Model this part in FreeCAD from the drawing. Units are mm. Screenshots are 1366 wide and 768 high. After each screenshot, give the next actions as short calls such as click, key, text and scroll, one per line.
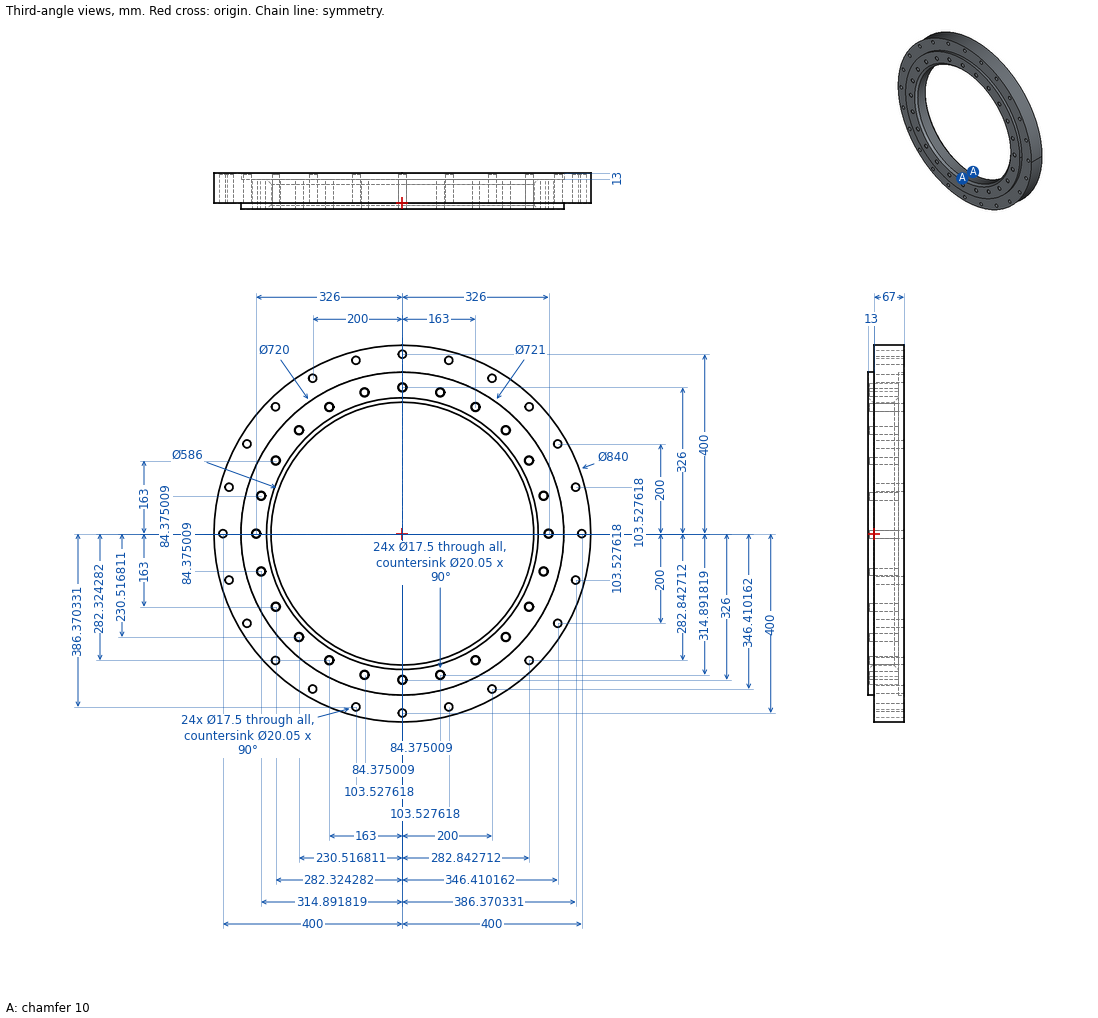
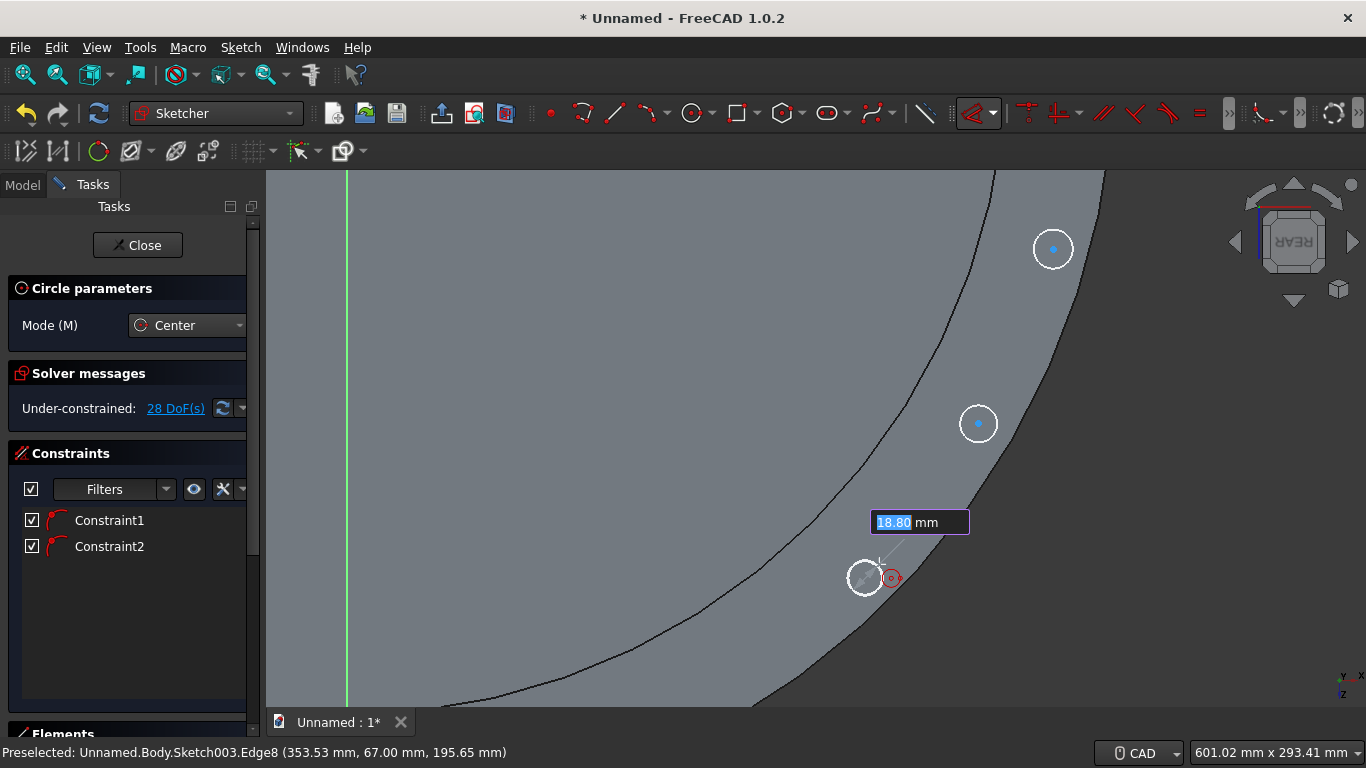
click(876, 561)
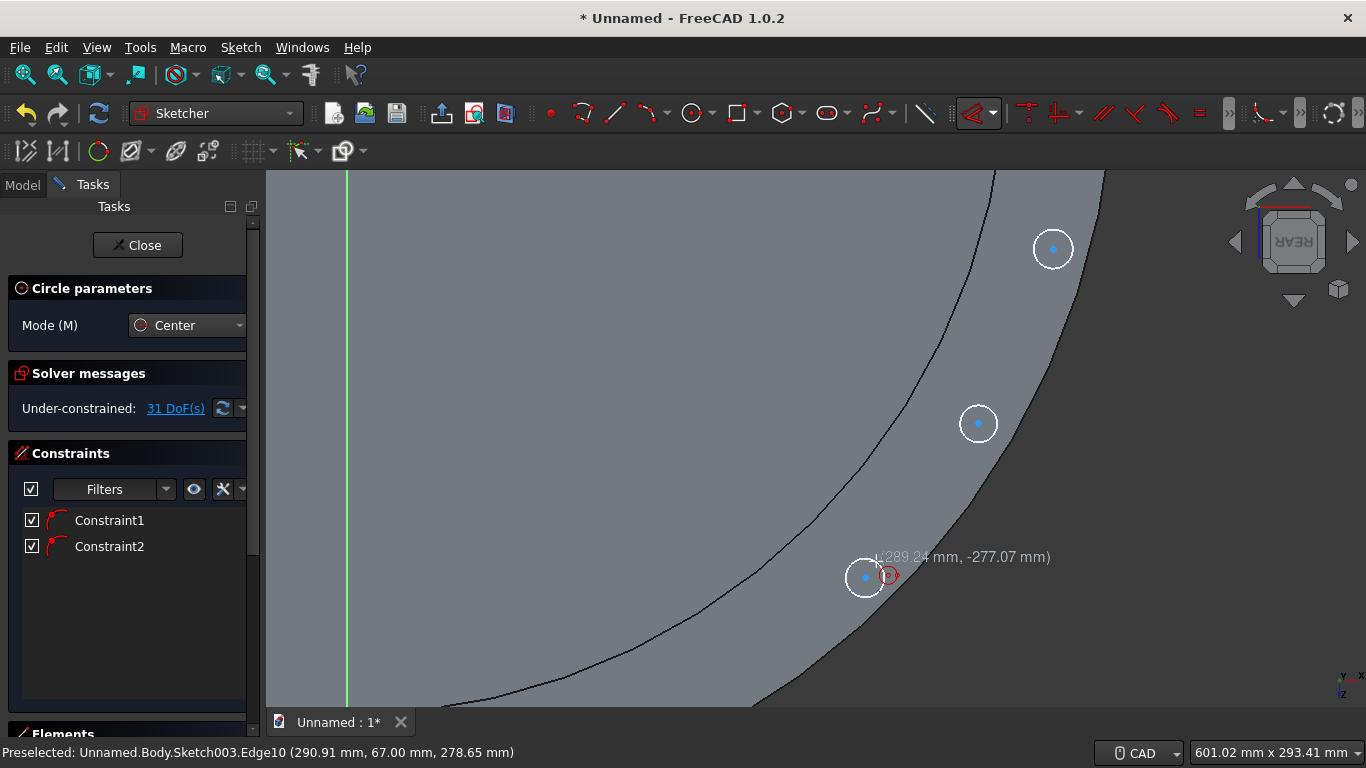
scroll(879, 564, down, 7)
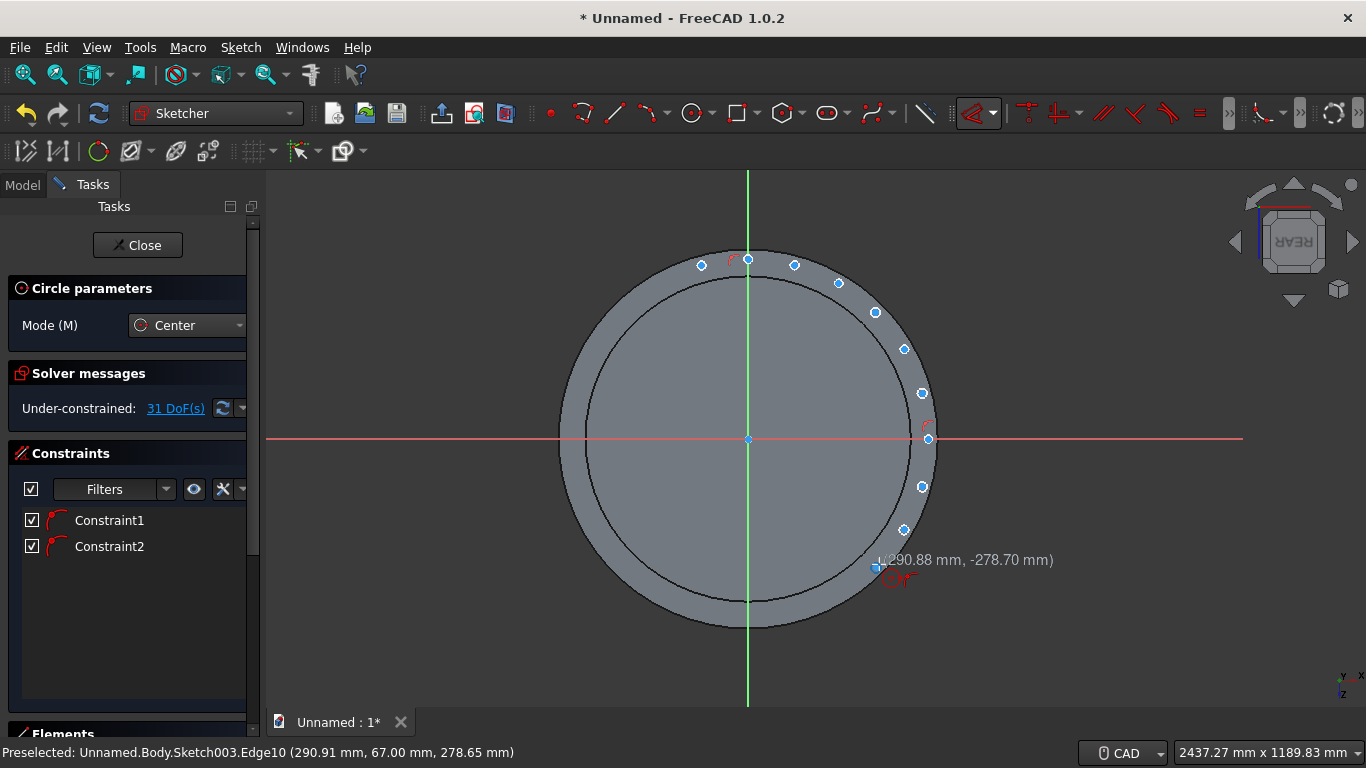
scroll(838, 595, up, 9)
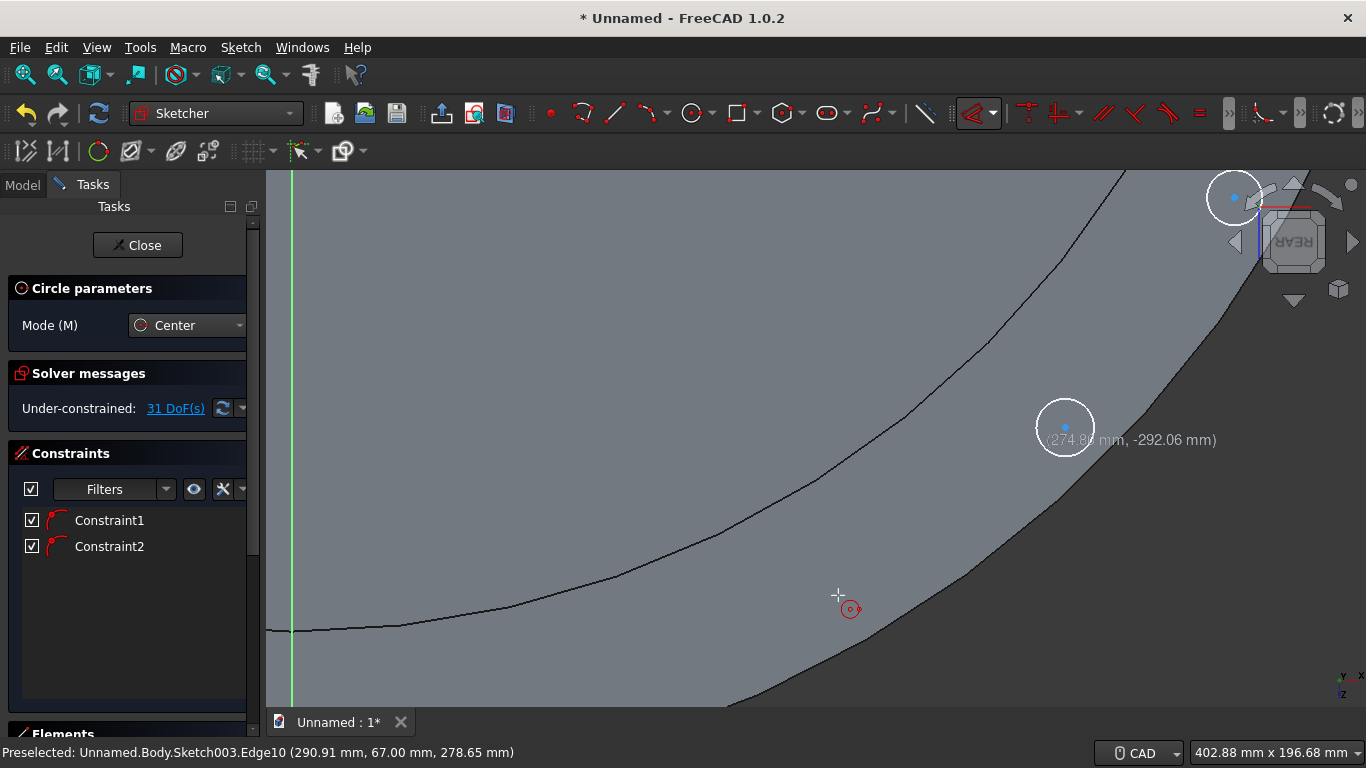
scroll(838, 595, down, 9)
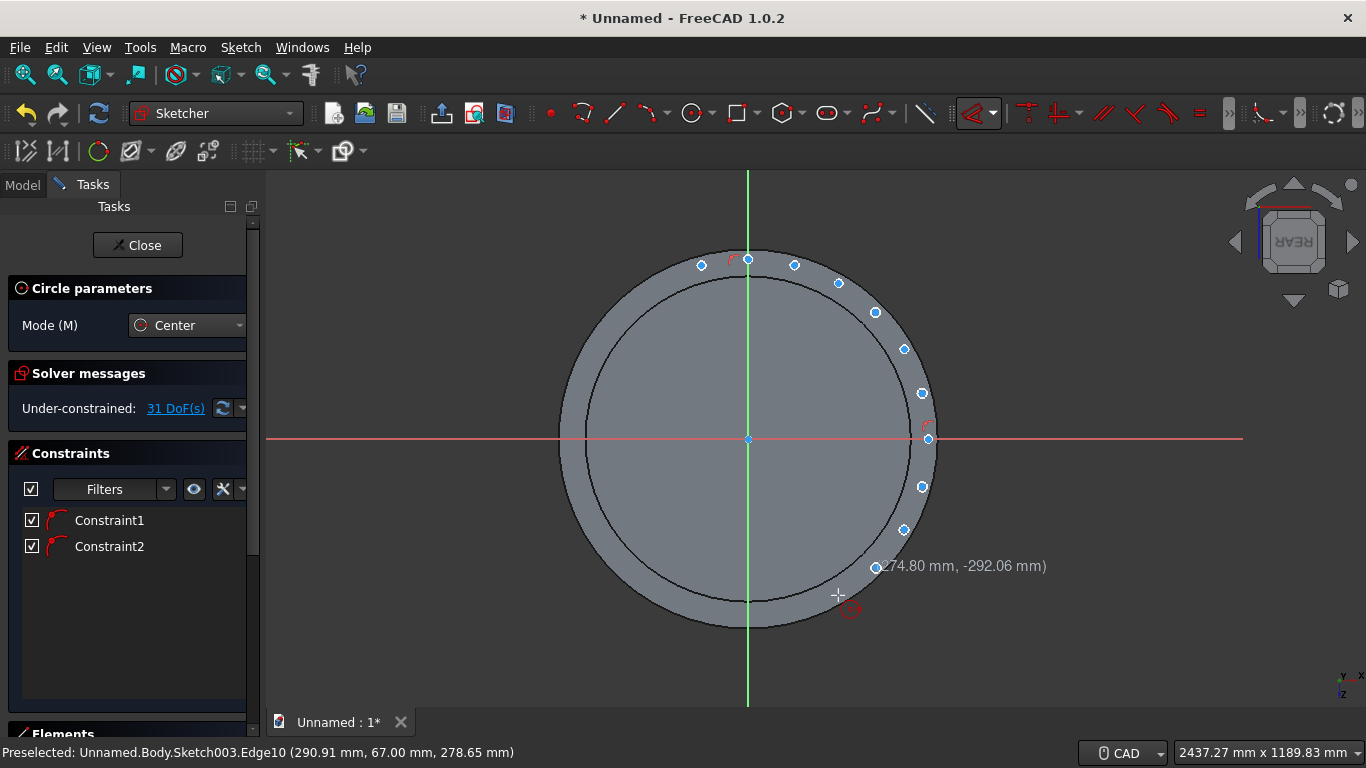
click(838, 595)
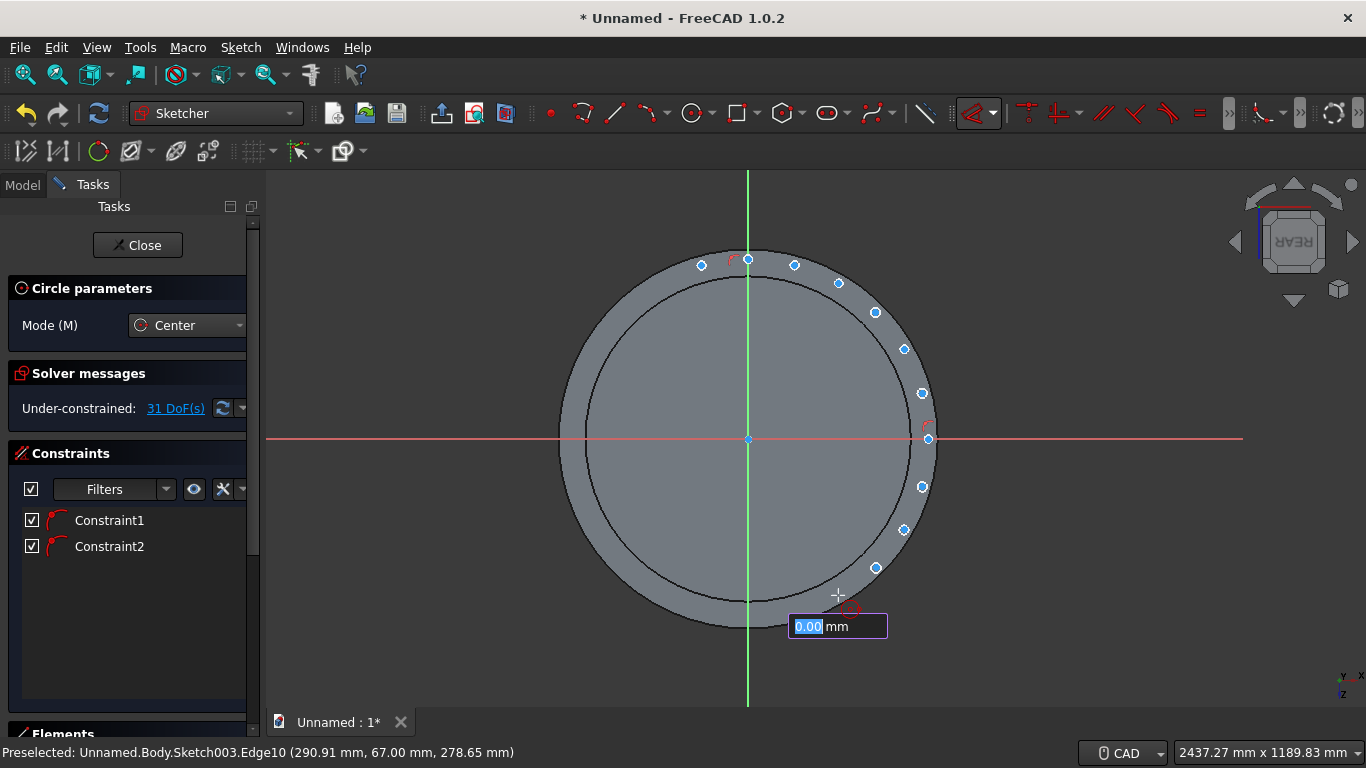
scroll(841, 593, up, 7)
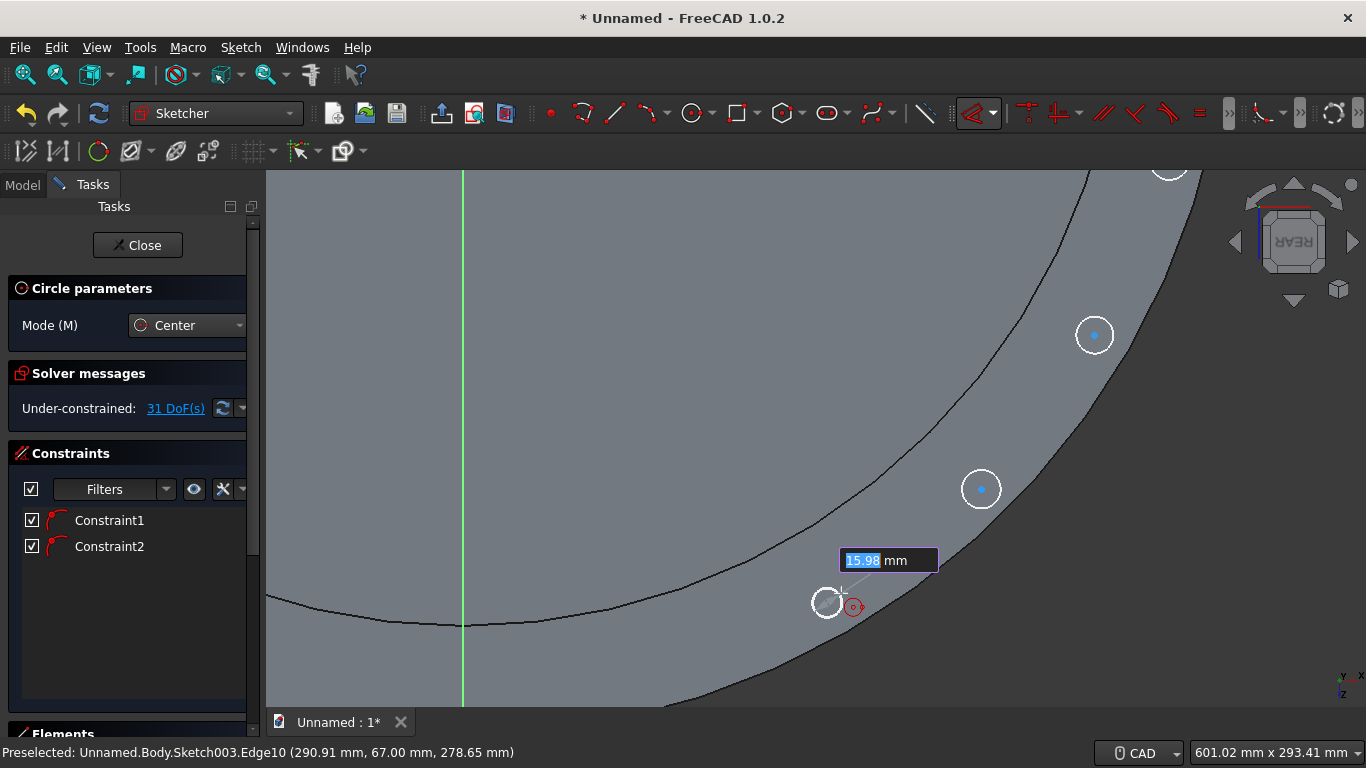
click(840, 589)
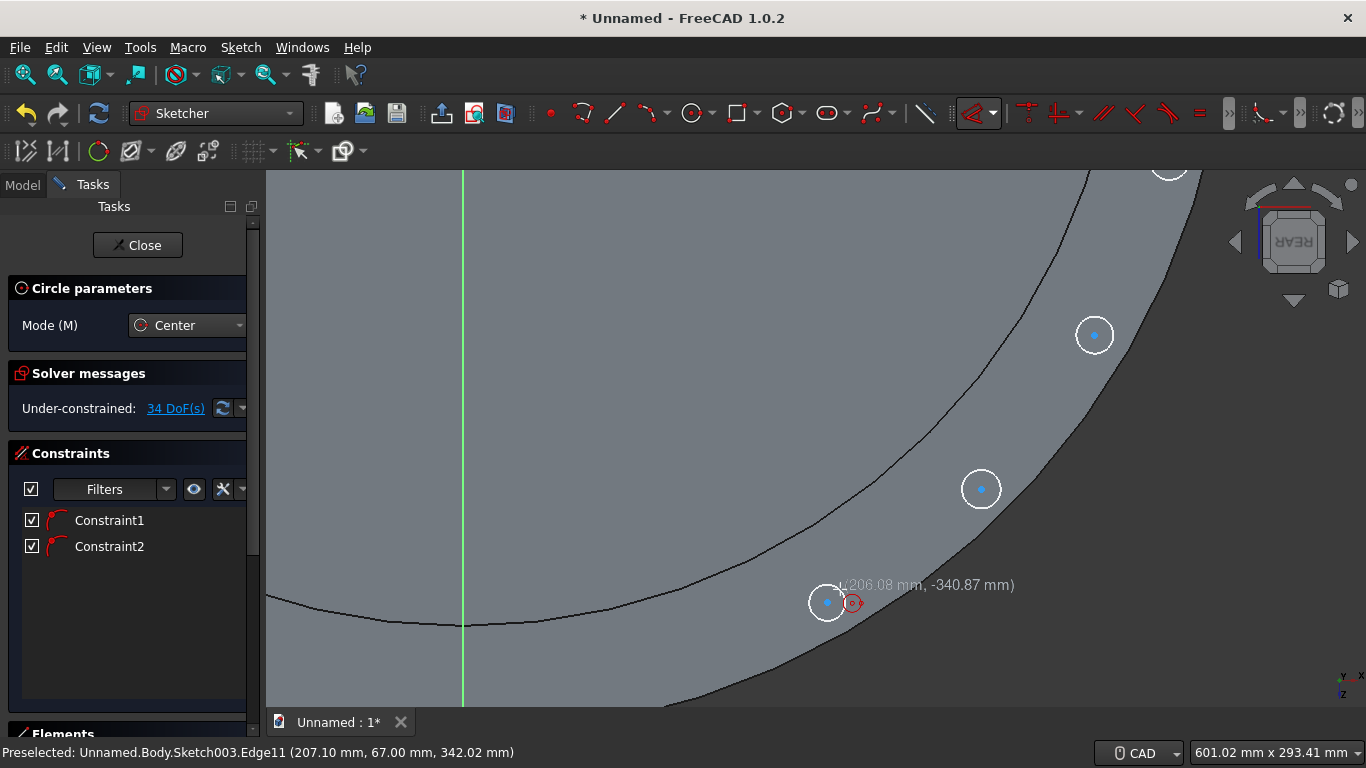
scroll(652, 673, up, 2)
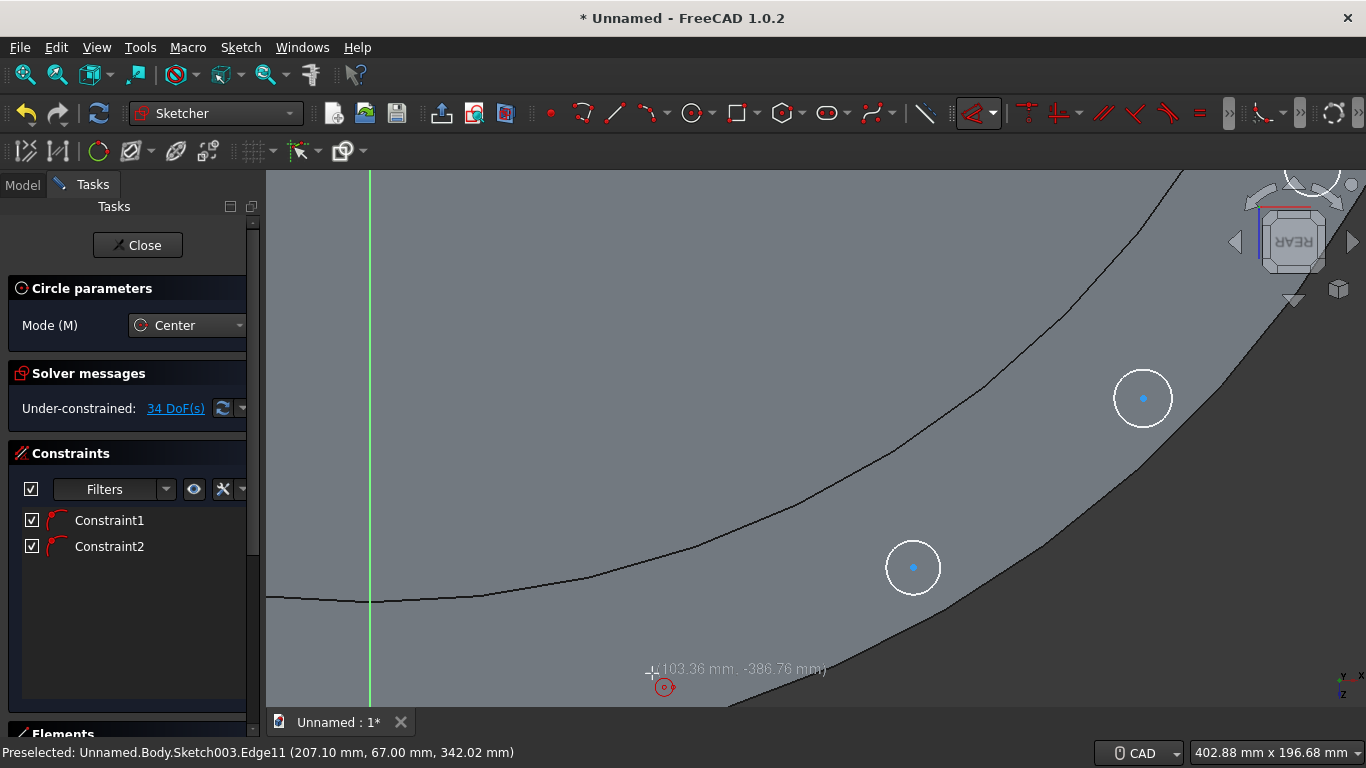
scroll(822, 601, down, 9)